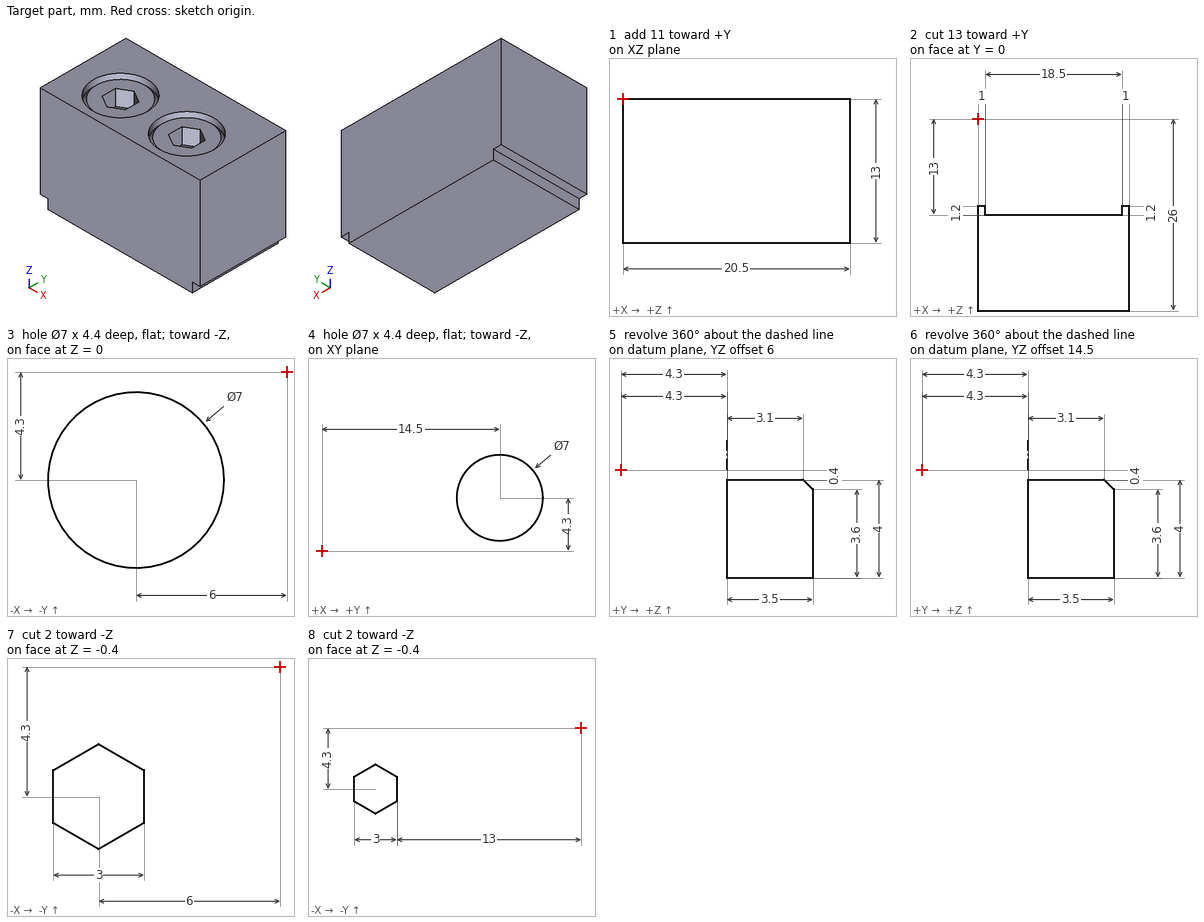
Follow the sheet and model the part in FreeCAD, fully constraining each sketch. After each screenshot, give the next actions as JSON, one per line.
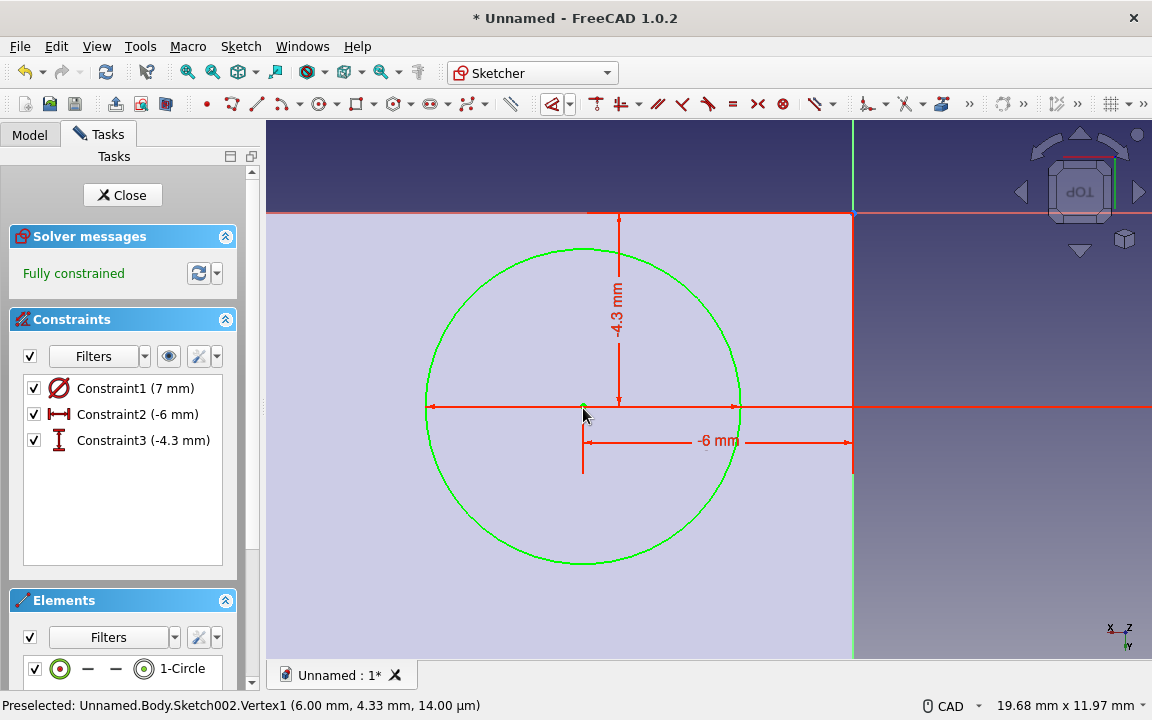
{"action": "left_click", "coordinate": [123, 195]}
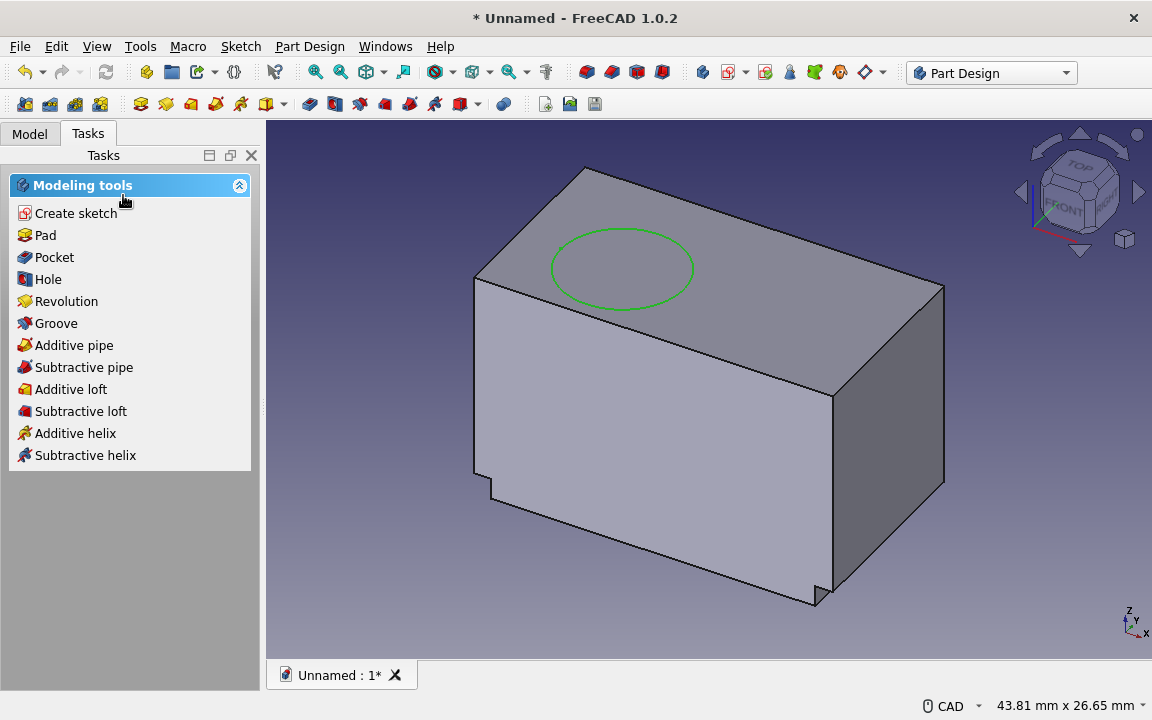
{"action": "left_click", "coordinate": [335, 104]}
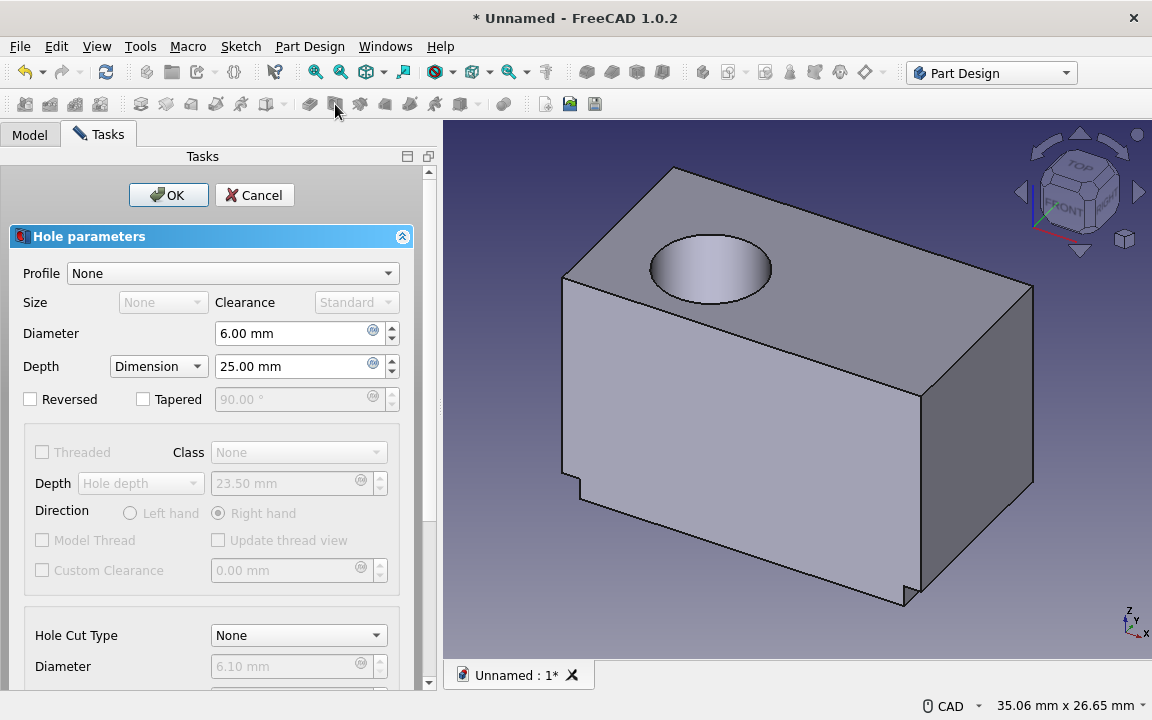
{"action": "triple_click", "coordinate": [300, 334]}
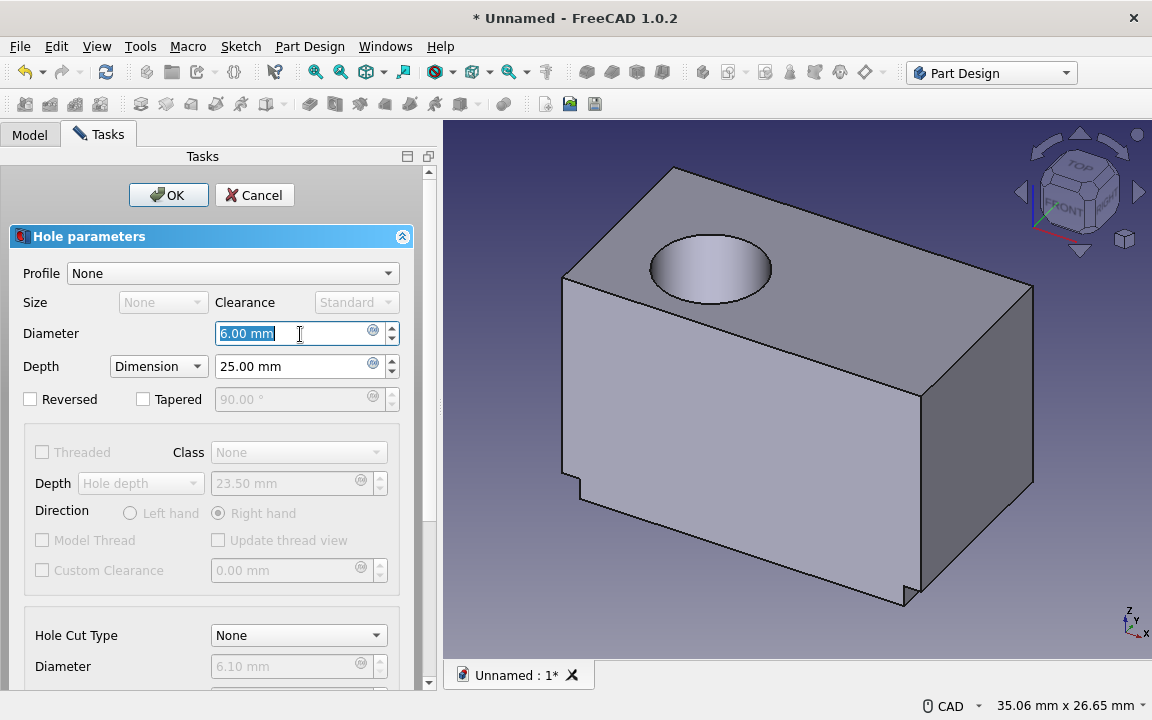
{"action": "type", "text": "7"}
{"action": "key", "text": "Tab"}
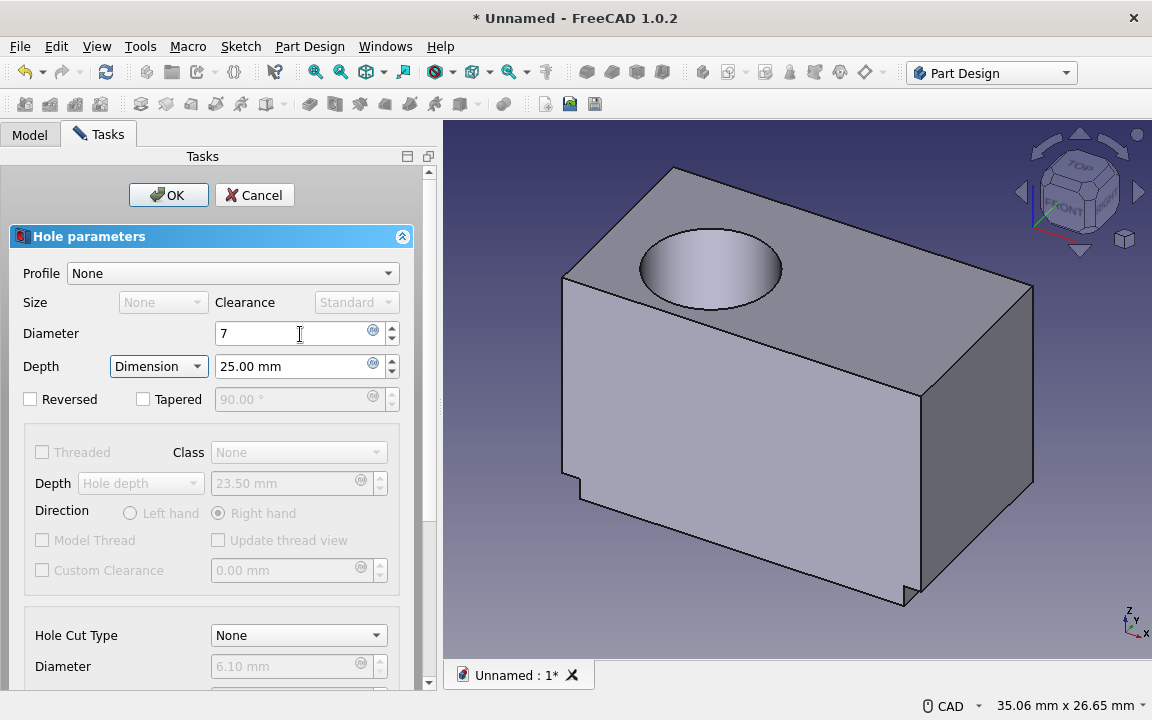
{"action": "triple_click", "coordinate": [300, 366]}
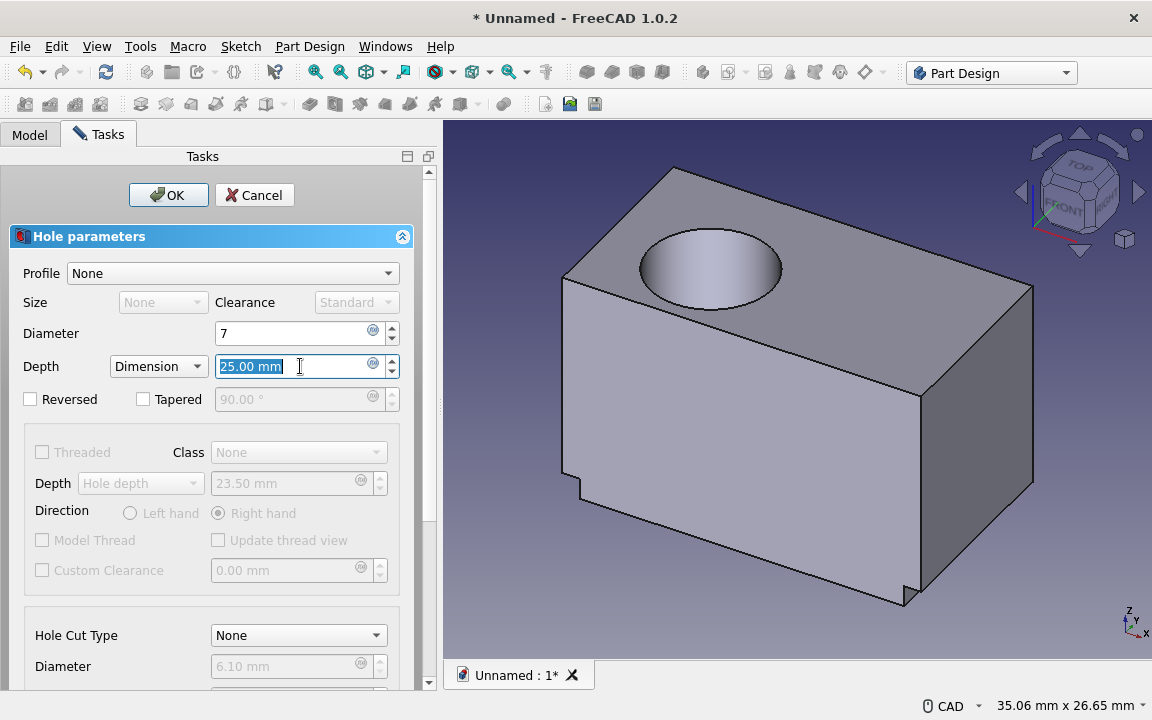
{"action": "type", "text": "4.4"}
{"action": "key", "text": "Tab"}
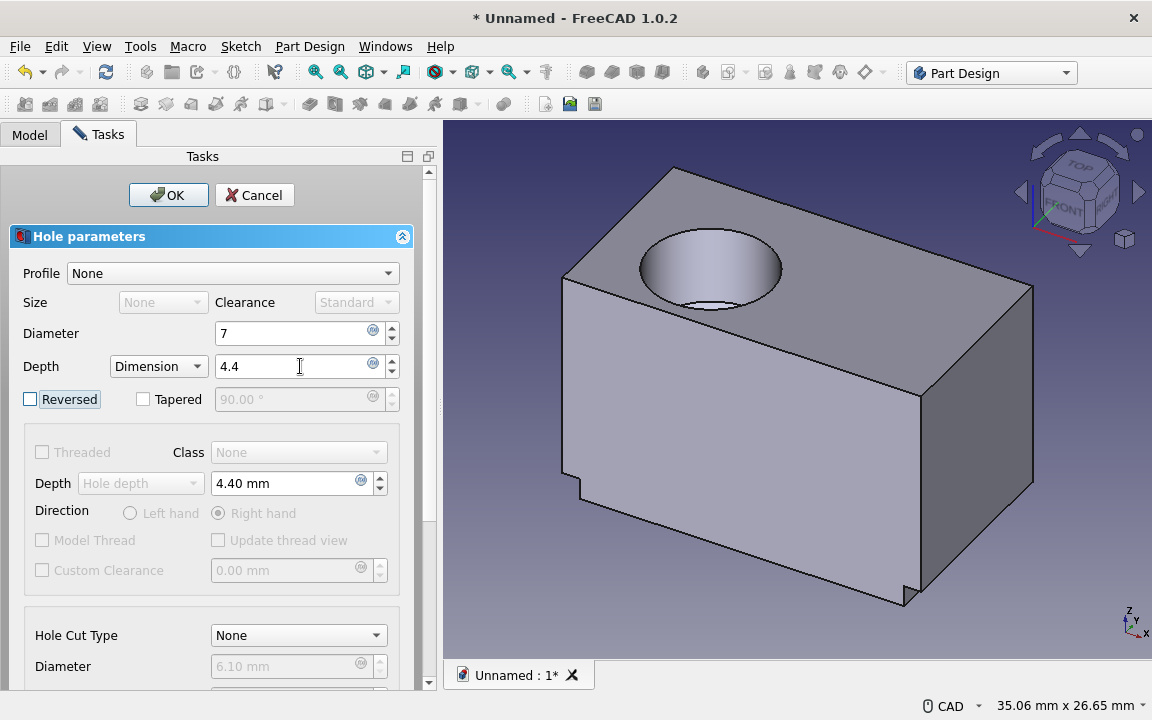
{"action": "scroll", "coordinate": [429, 428], "scroll_direction": "down", "scroll_amount": 4}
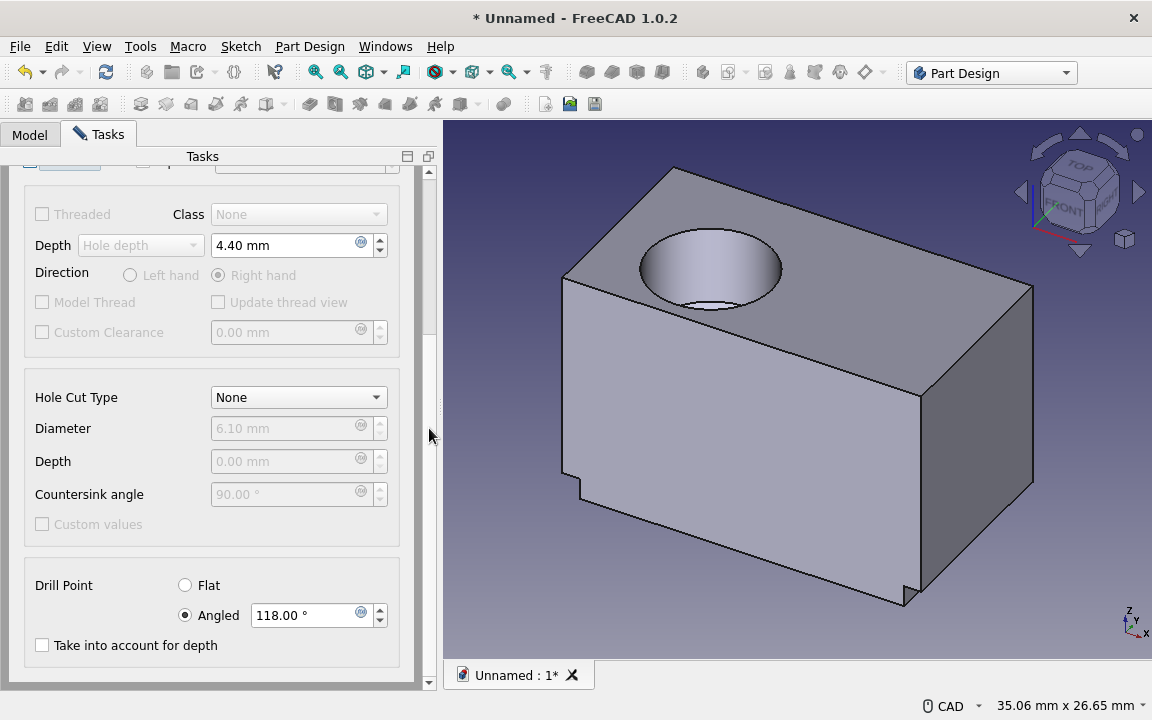
{"action": "left_click", "coordinate": [186, 583]}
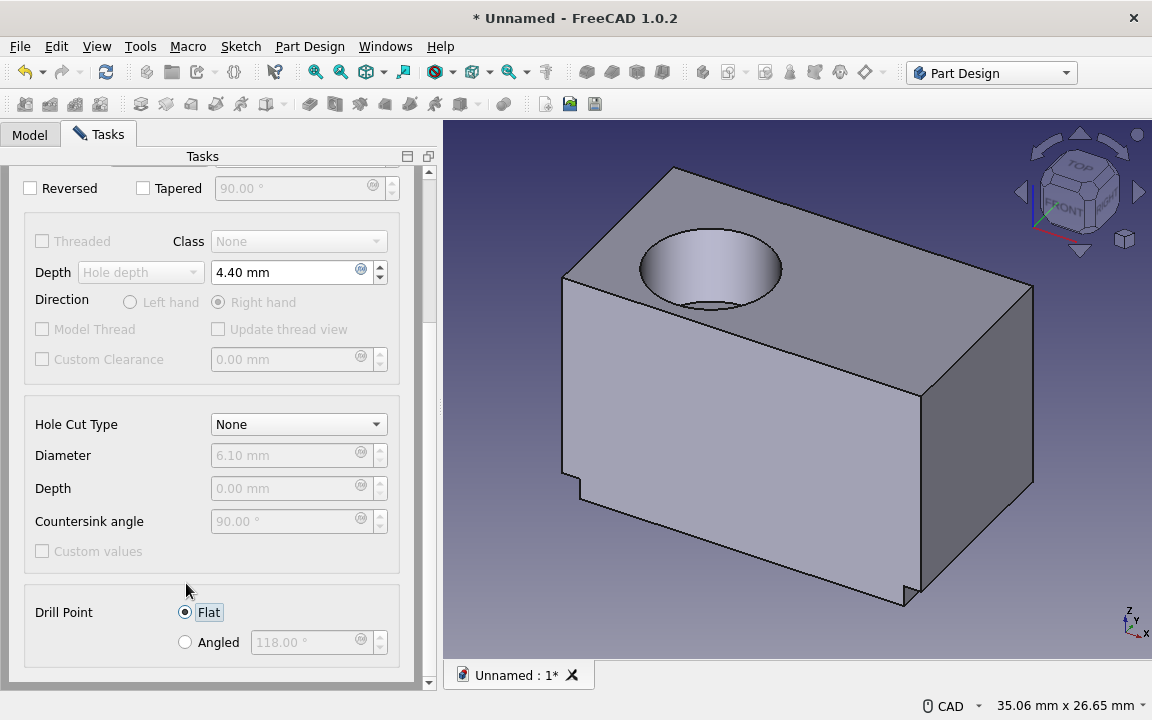
{"action": "scroll", "coordinate": [429, 428], "scroll_direction": "up", "scroll_amount": 5}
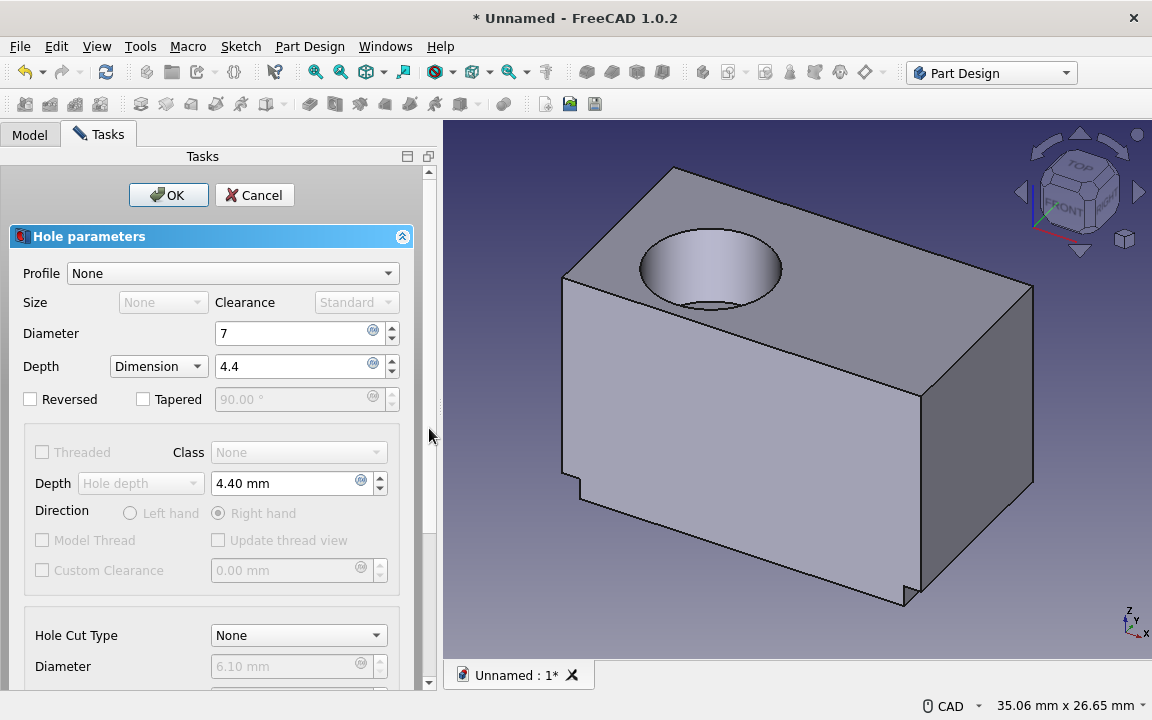
{"action": "left_click", "coordinate": [169, 195]}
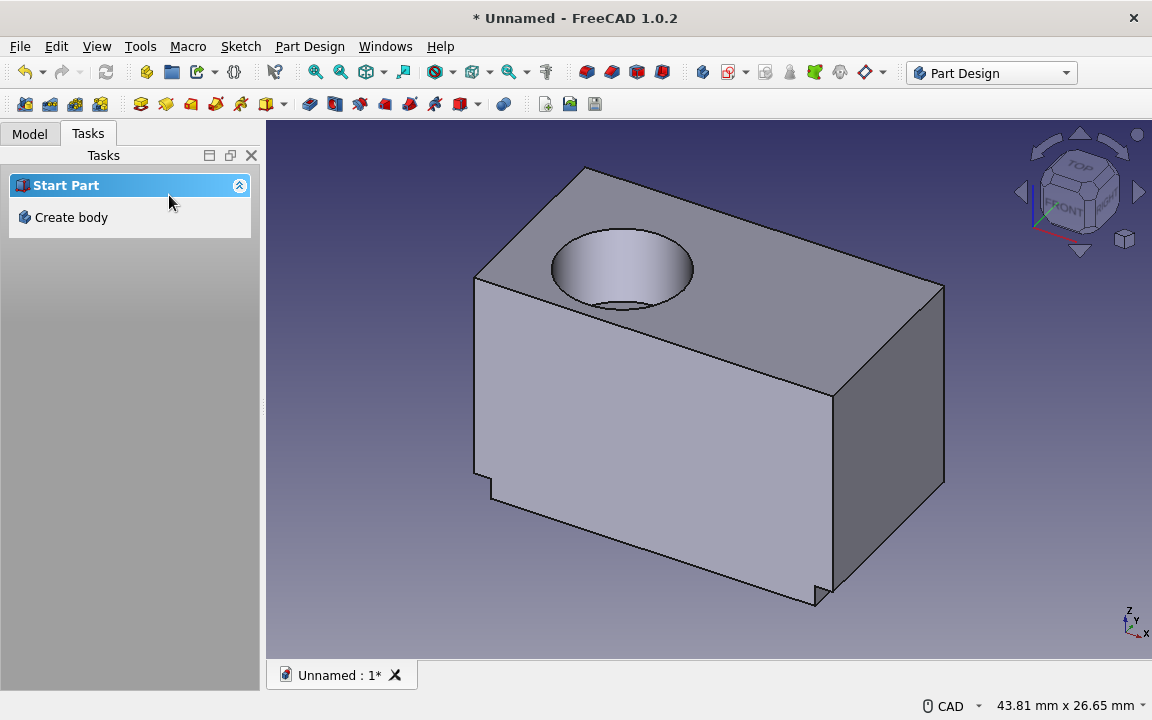
{"action": "left_click", "coordinate": [728, 72]}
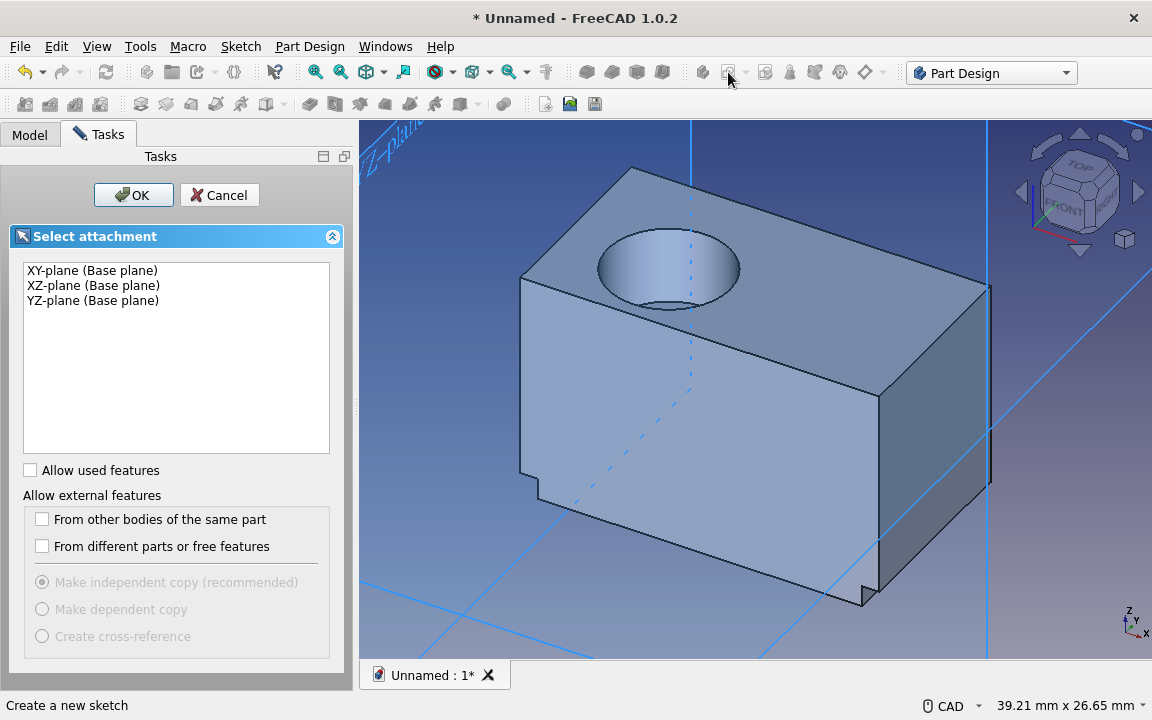
{"action": "left_click", "coordinate": [84, 270]}